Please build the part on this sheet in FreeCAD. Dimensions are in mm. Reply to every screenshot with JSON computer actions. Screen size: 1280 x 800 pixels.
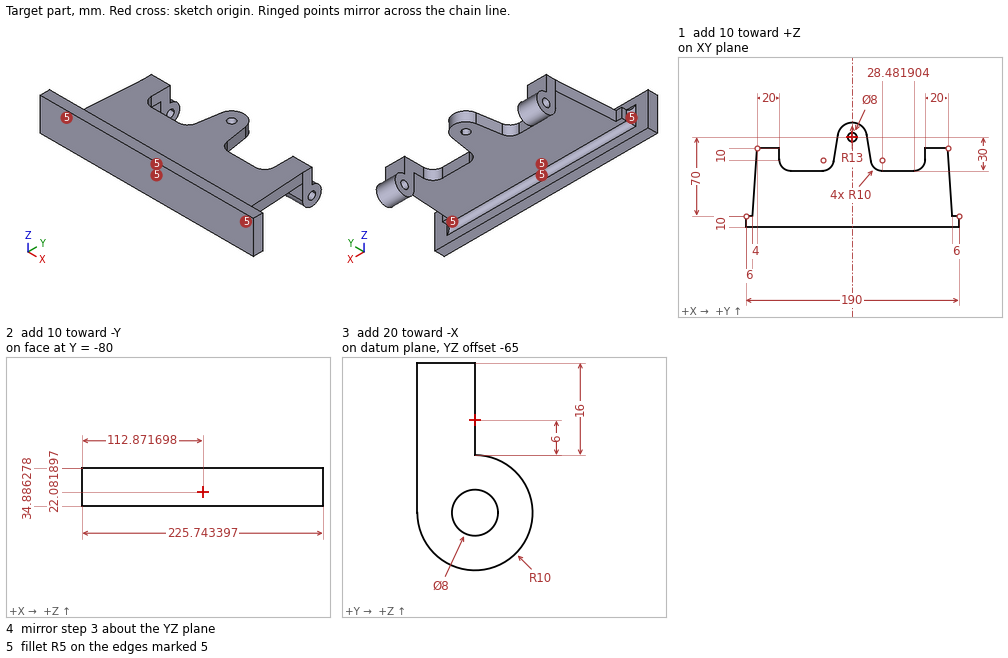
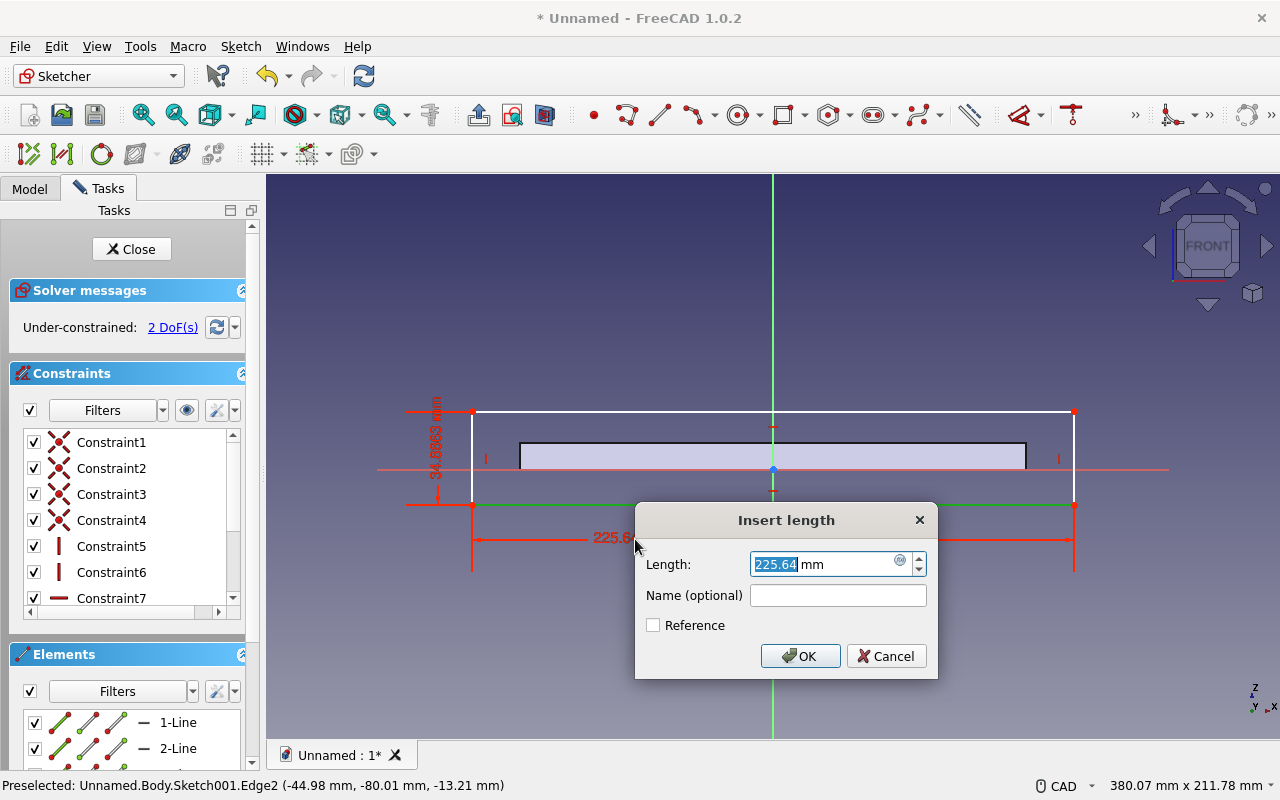
{"action": "type", "text": "225.743397"}
{"action": "key", "text": "Return"}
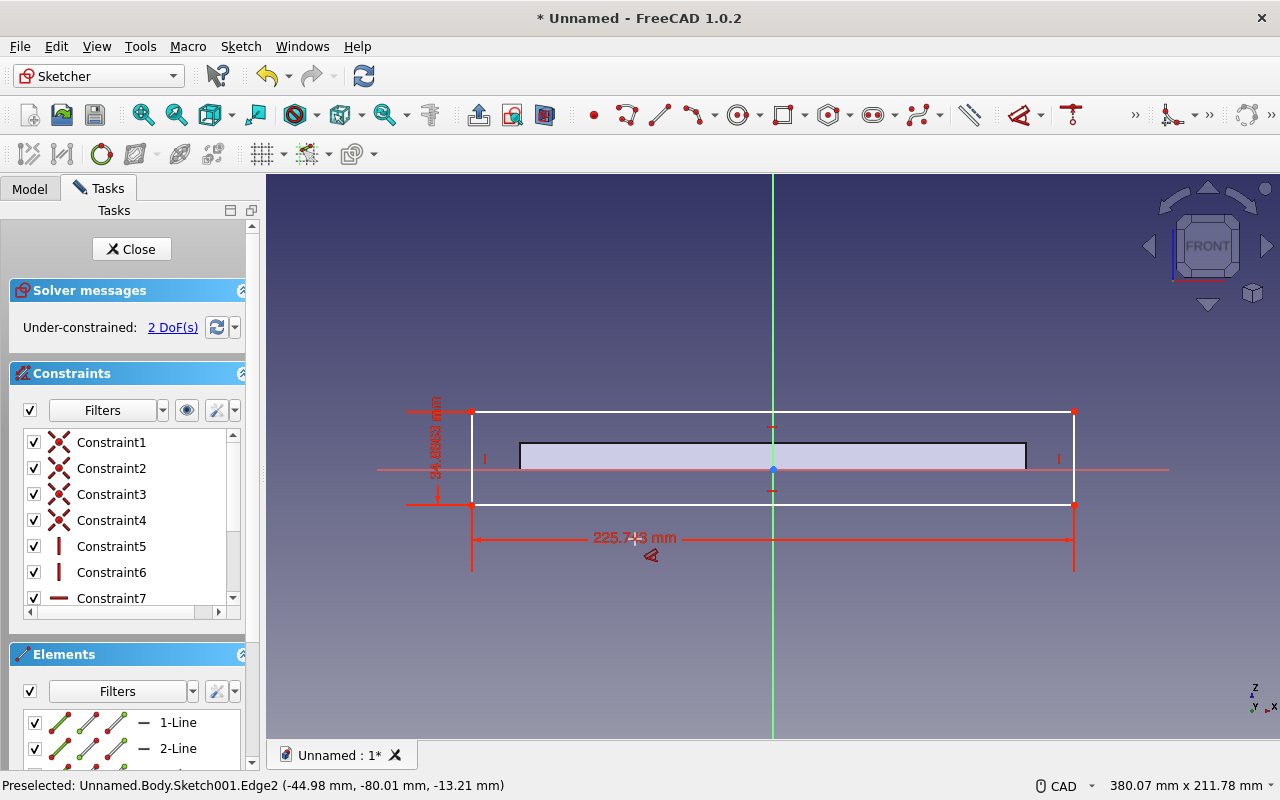
{"action": "left_click", "coordinate": [472, 412]}
{"action": "left_click", "coordinate": [807, 441]}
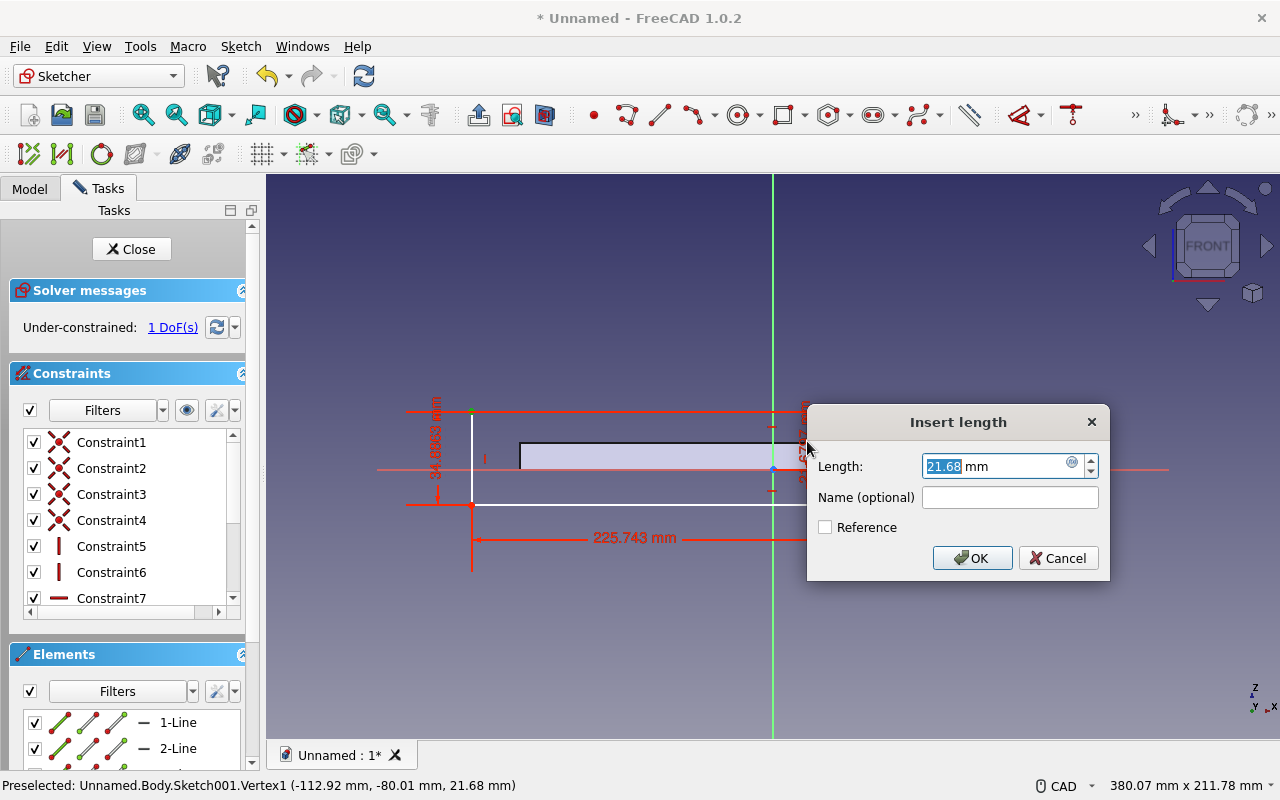
{"action": "type", "text": "22.081897"}
{"action": "key", "text": "Return"}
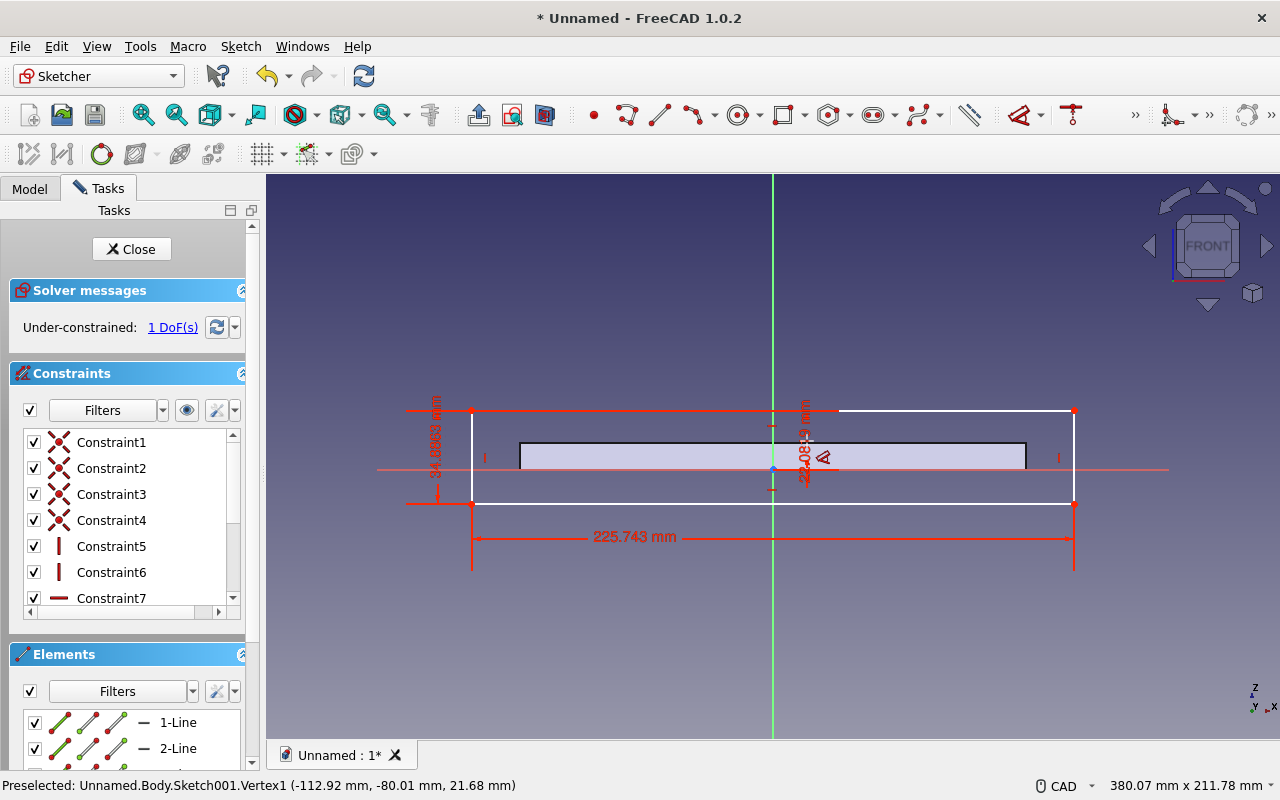
{"action": "left_click", "coordinate": [472, 411]}
{"action": "left_click", "coordinate": [622, 377]}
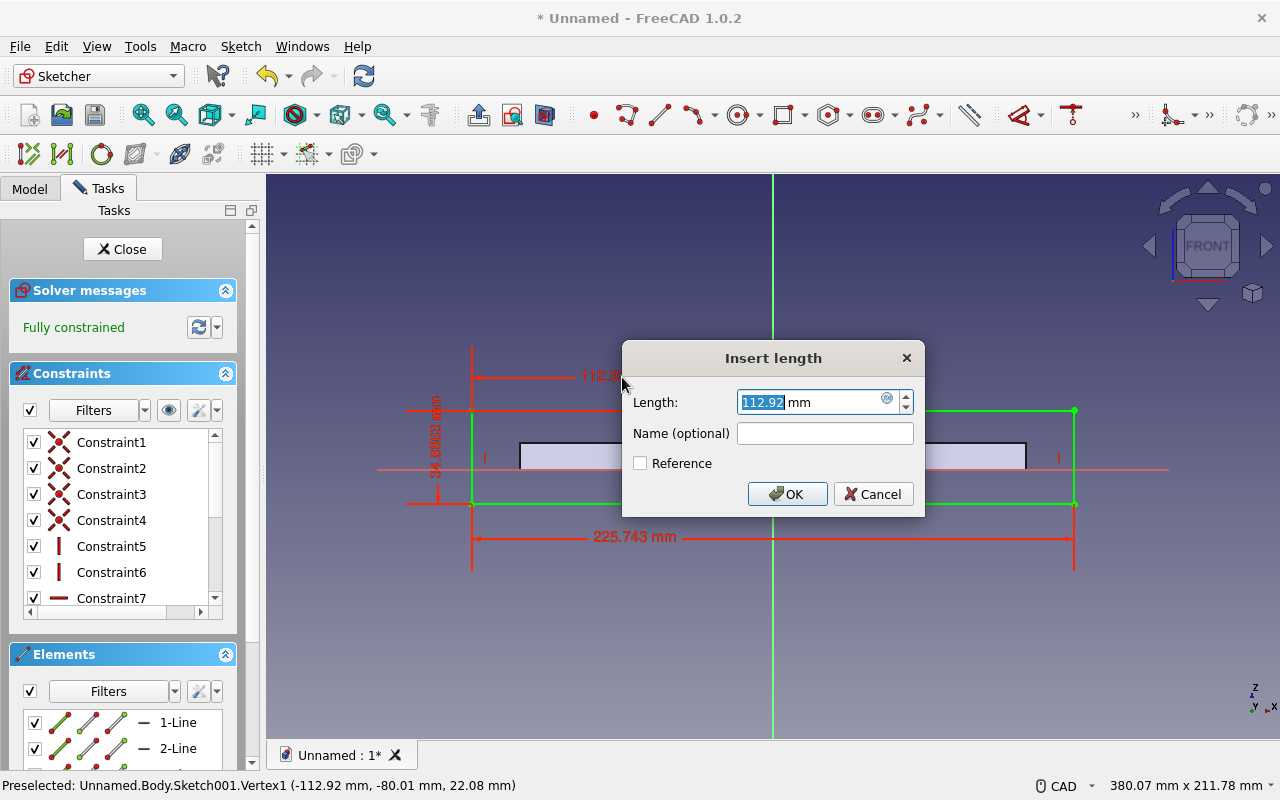
{"action": "type", "text": "112.871698"}
{"action": "key", "text": "Return"}
{"action": "key", "text": "Escape"}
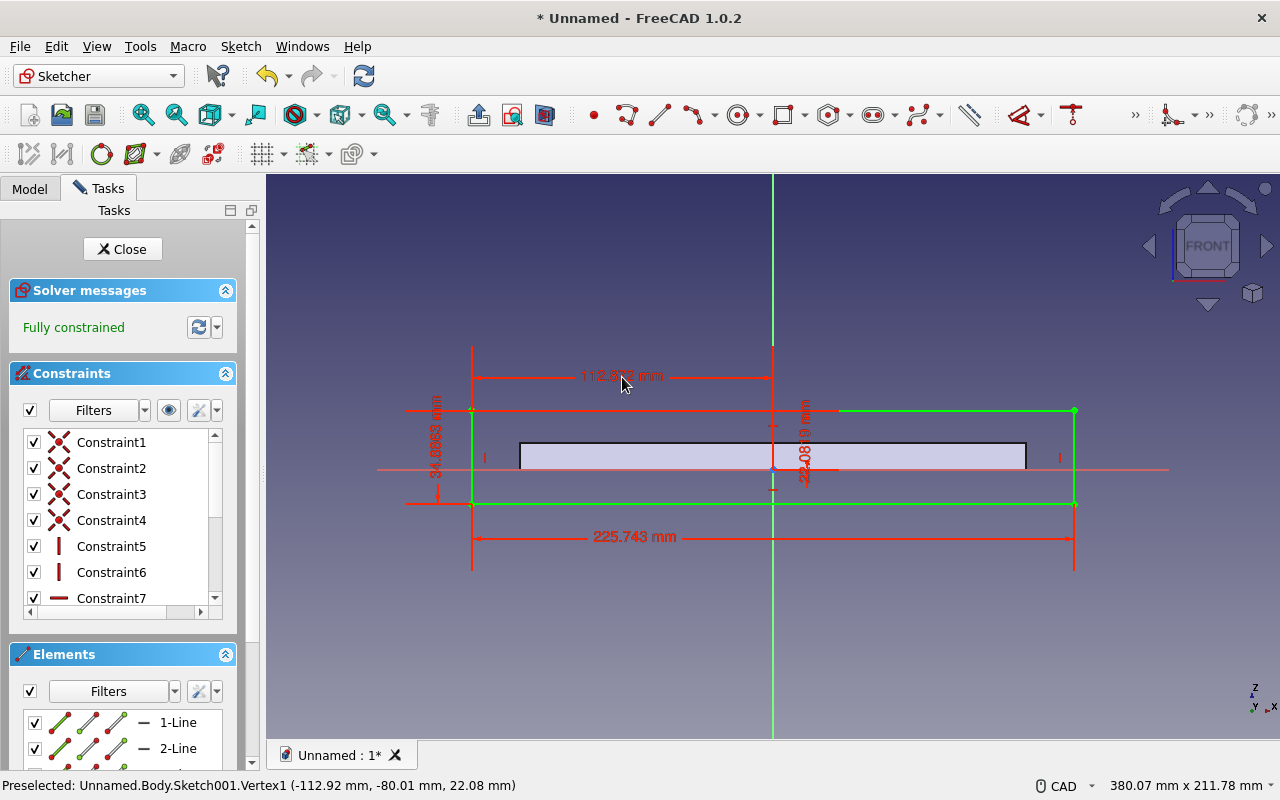
{"action": "left_click", "coordinate": [123, 249]}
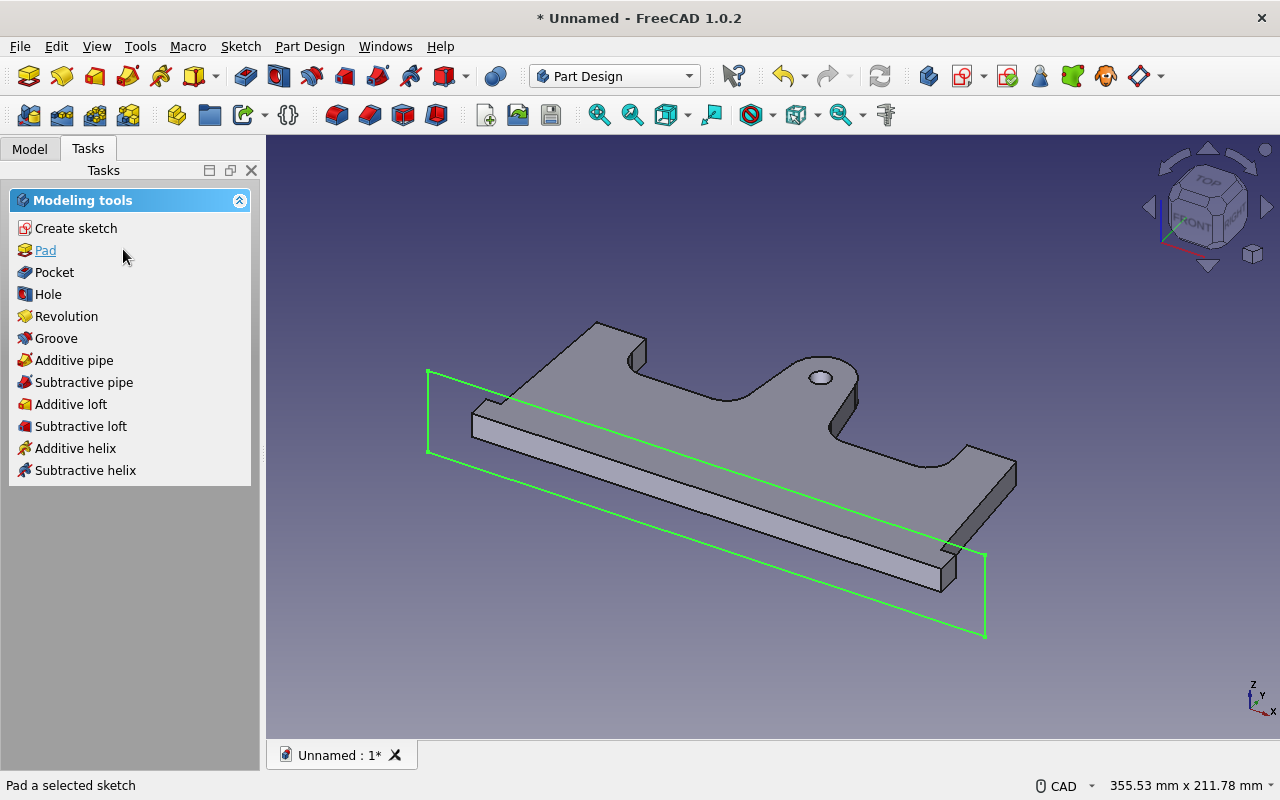
{"action": "left_click", "coordinate": [29, 76]}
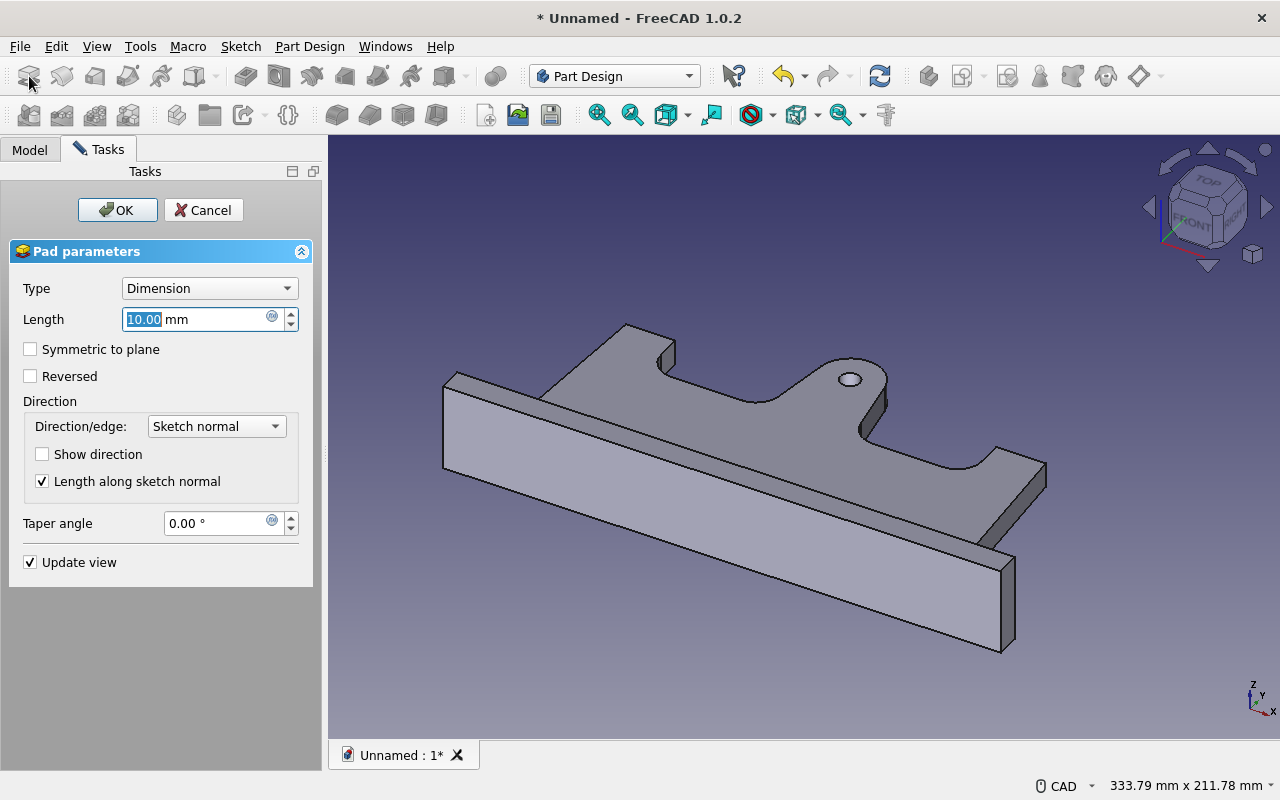
{"action": "type", "text": "10"}
{"action": "key", "text": "Tab"}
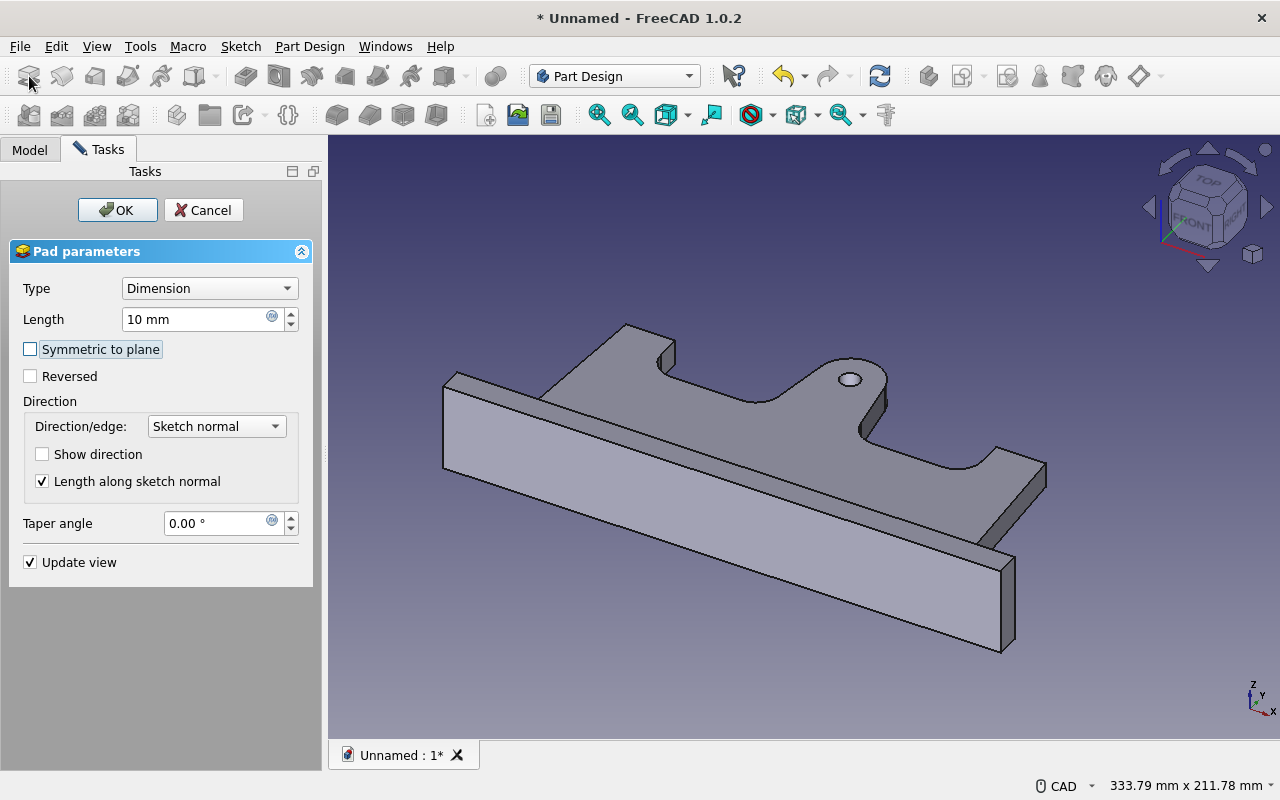
{"action": "left_click", "coordinate": [118, 210]}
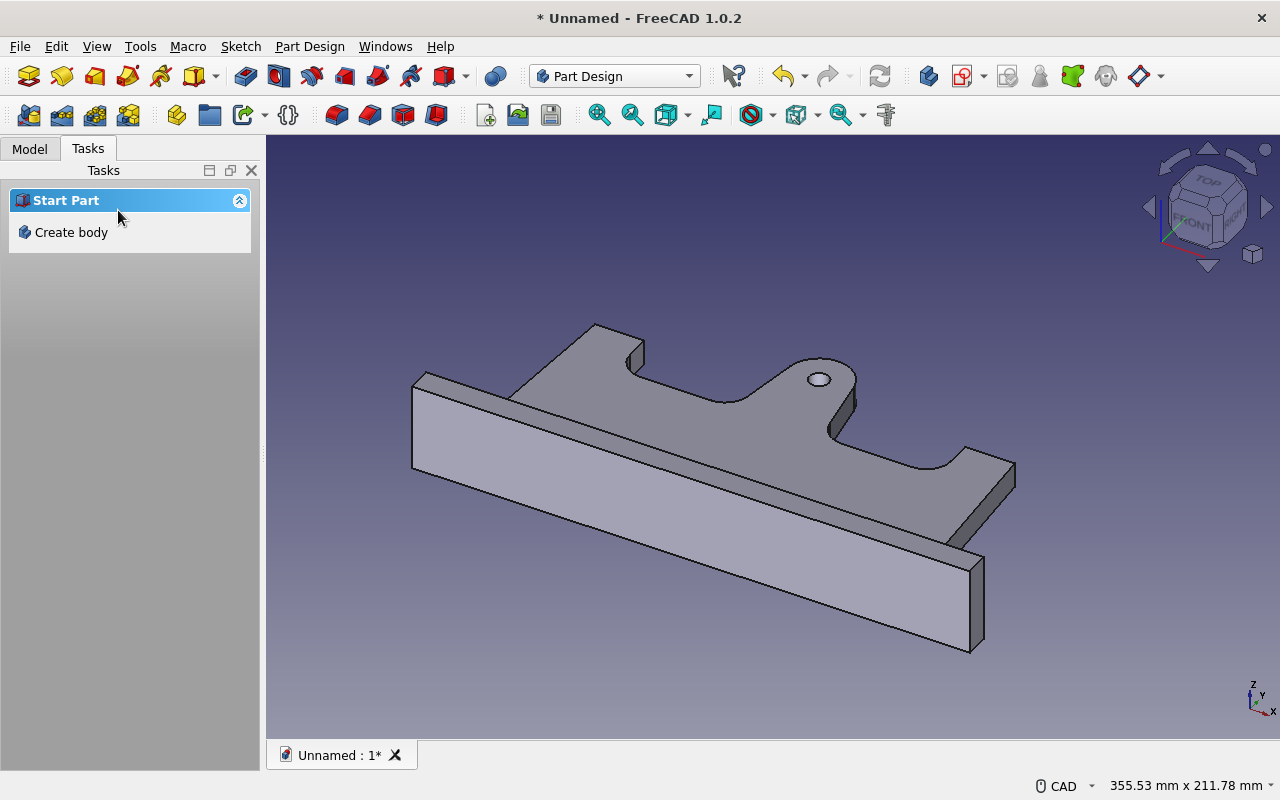
{"action": "left_click", "coordinate": [30, 148]}